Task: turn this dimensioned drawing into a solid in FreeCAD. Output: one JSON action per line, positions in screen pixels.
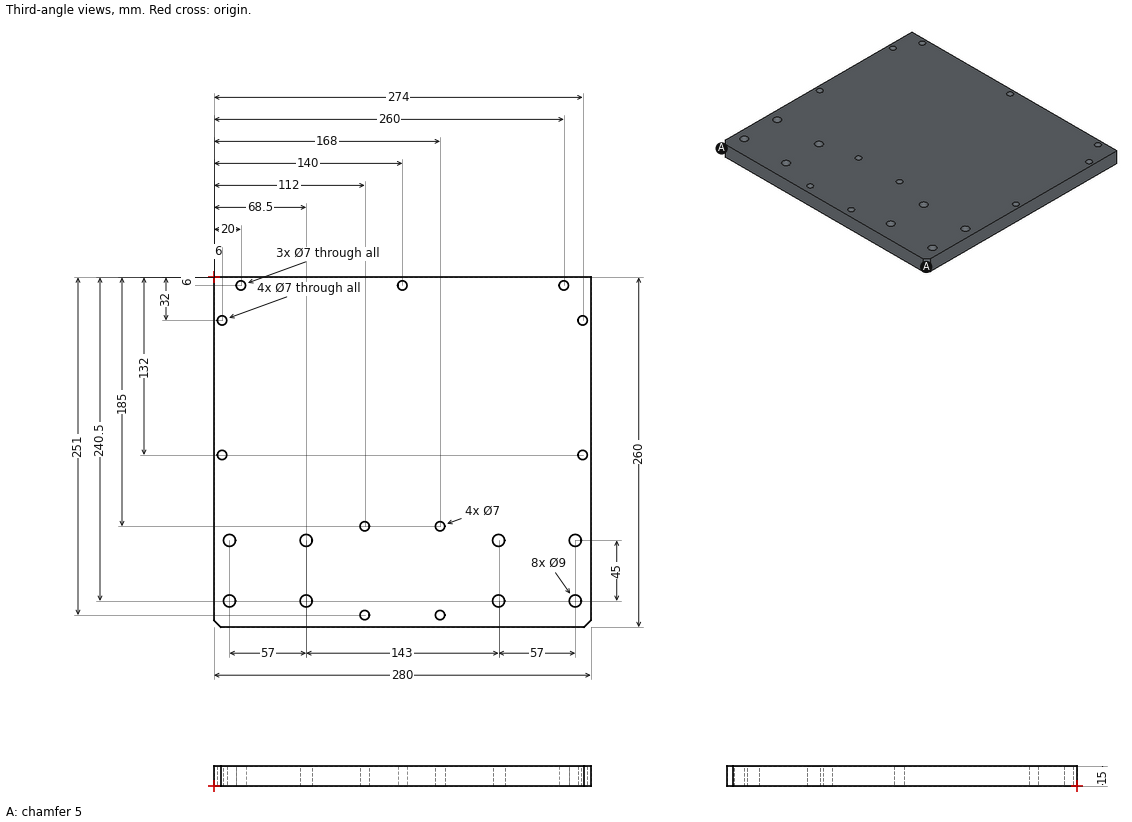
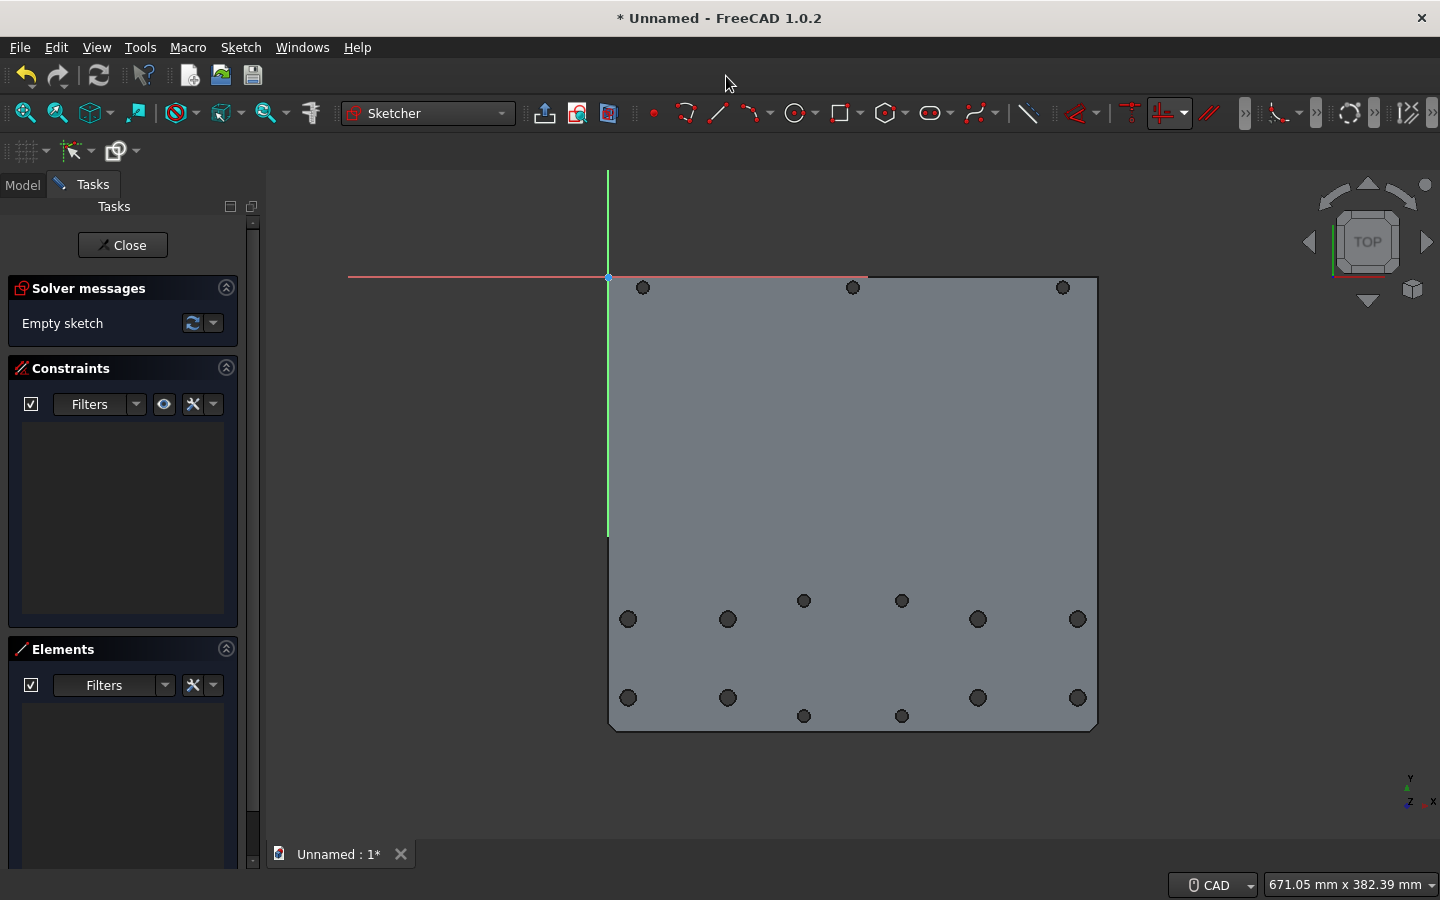
{"action": "scroll", "coordinate": [986, 198], "scroll_direction": "up", "scroll_amount": 2}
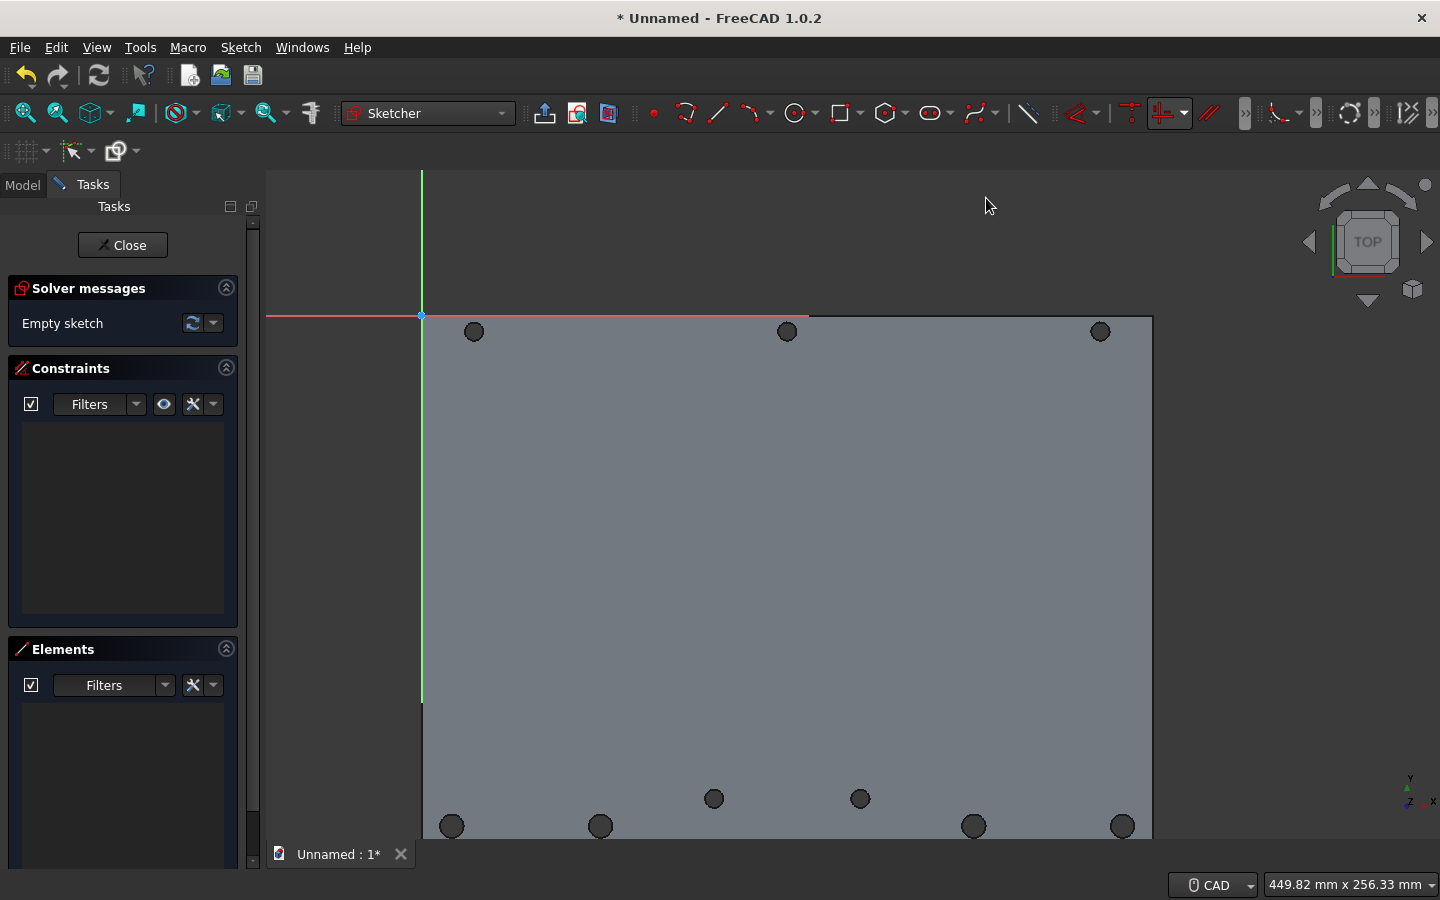
{"action": "left_click", "coordinate": [796, 114]}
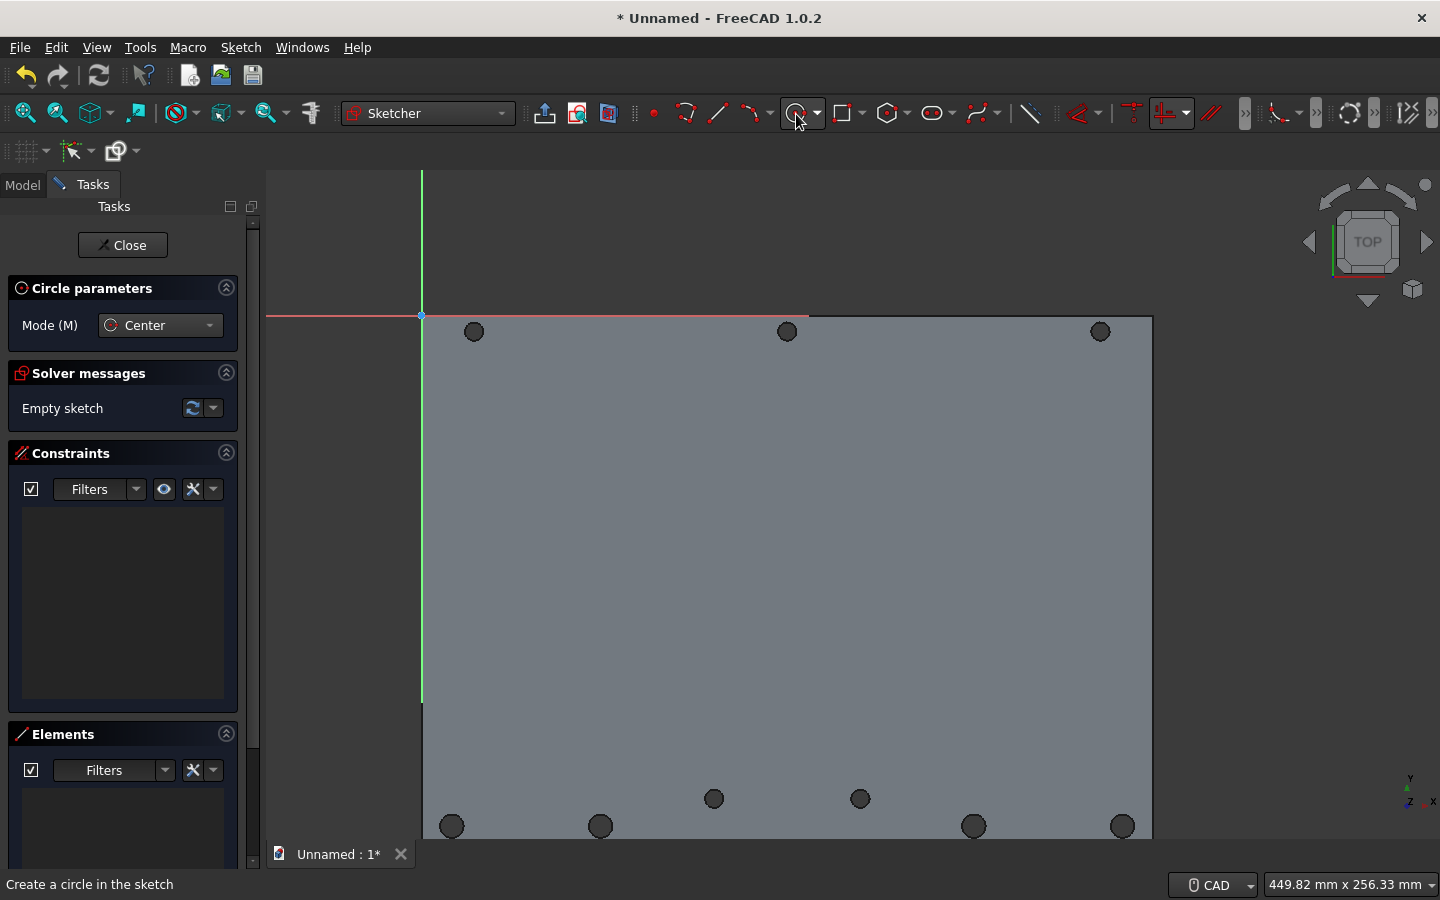
{"action": "scroll", "coordinate": [438, 399], "scroll_direction": "up", "scroll_amount": 5}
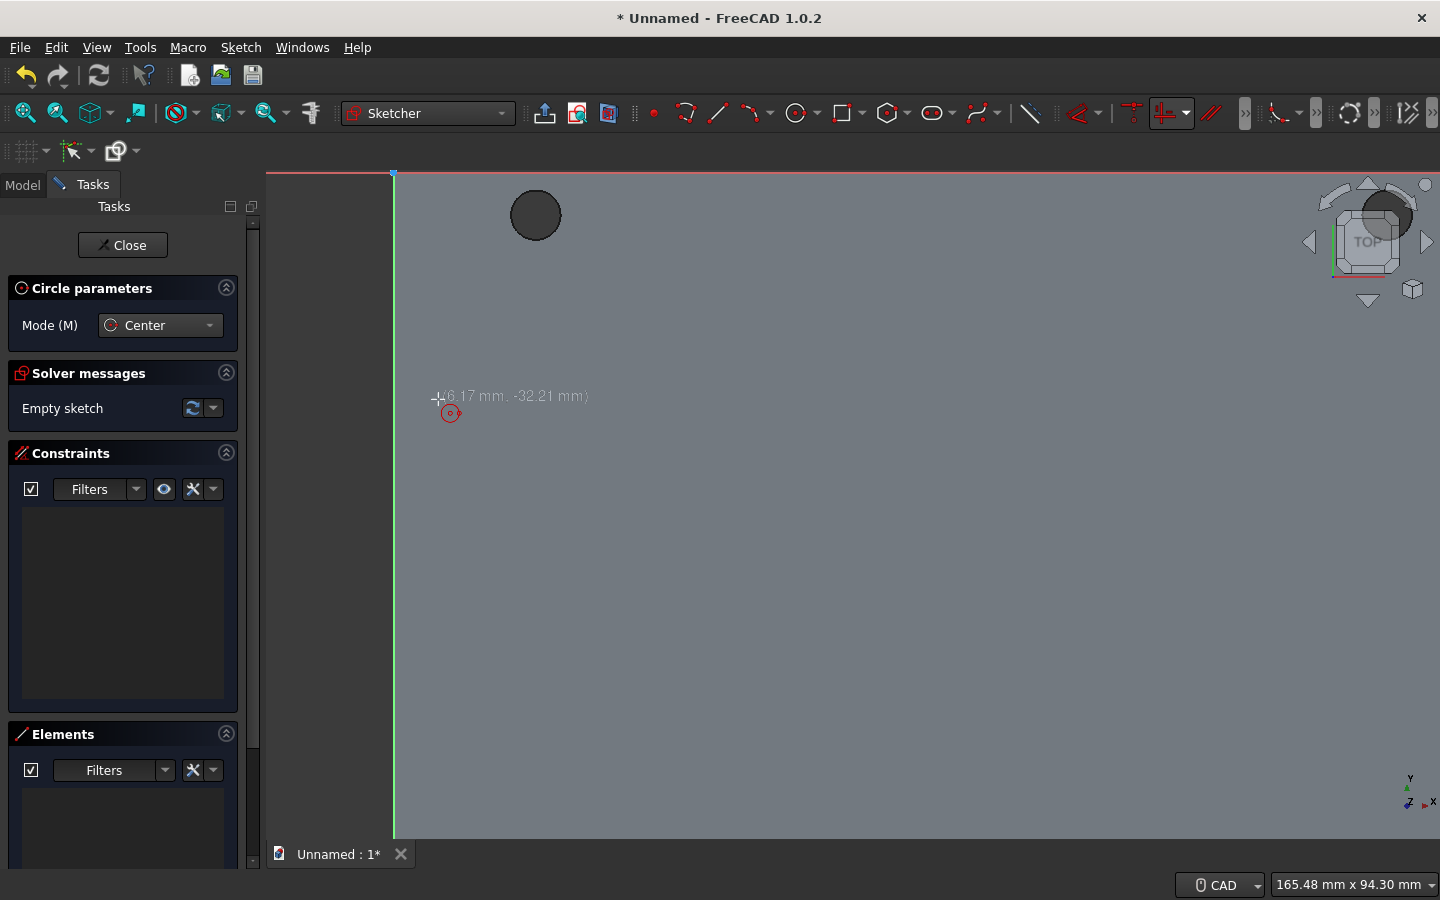
{"action": "left_click", "coordinate": [437, 400]}
{"action": "mouse_move", "coordinate": [454, 382]}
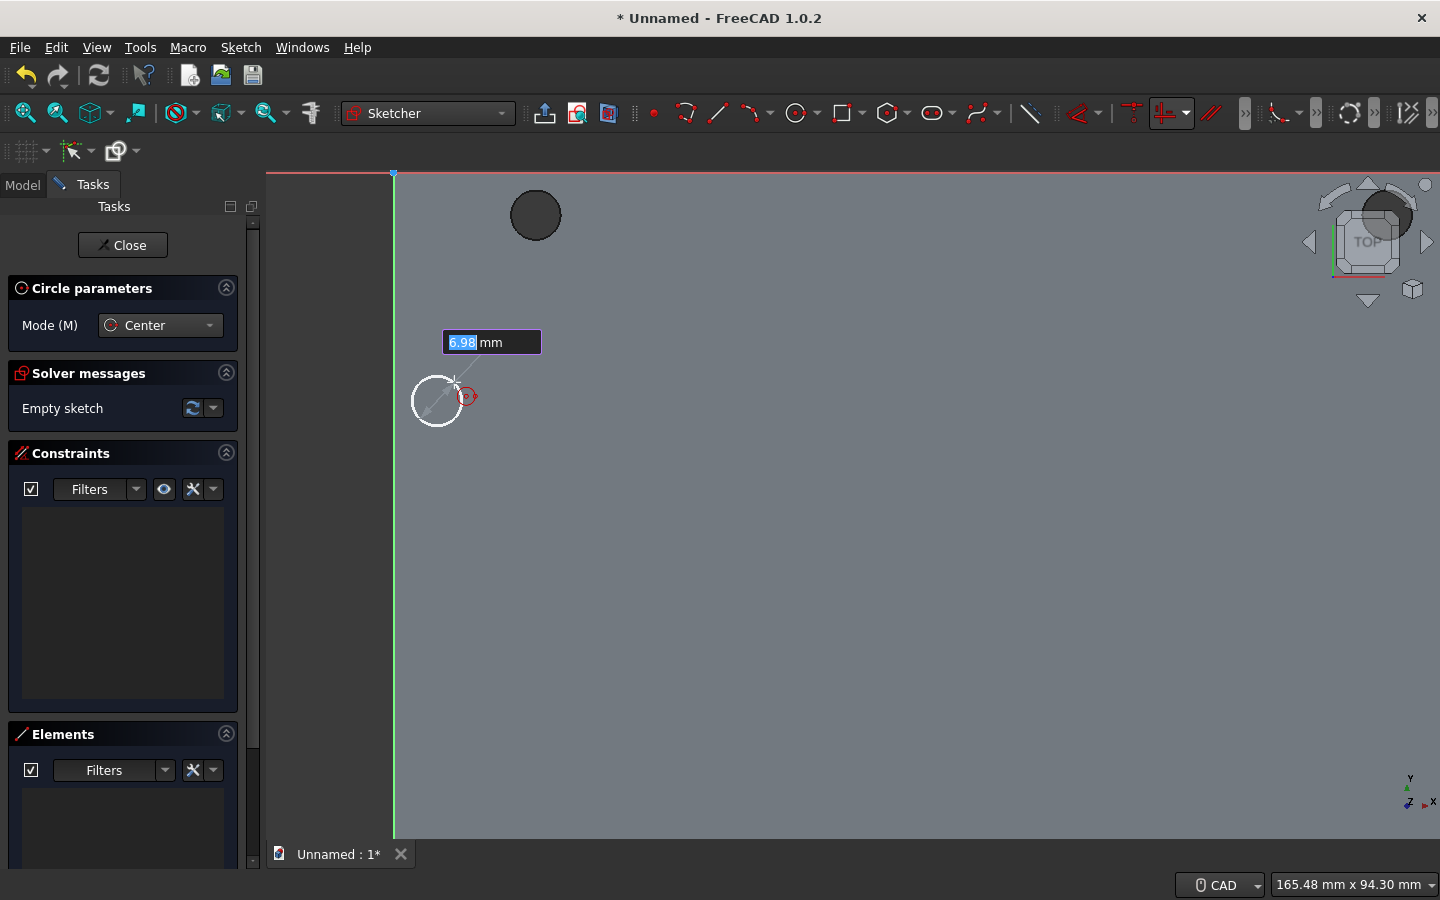
{"action": "type", "text": "7"}
{"action": "key", "text": "Return"}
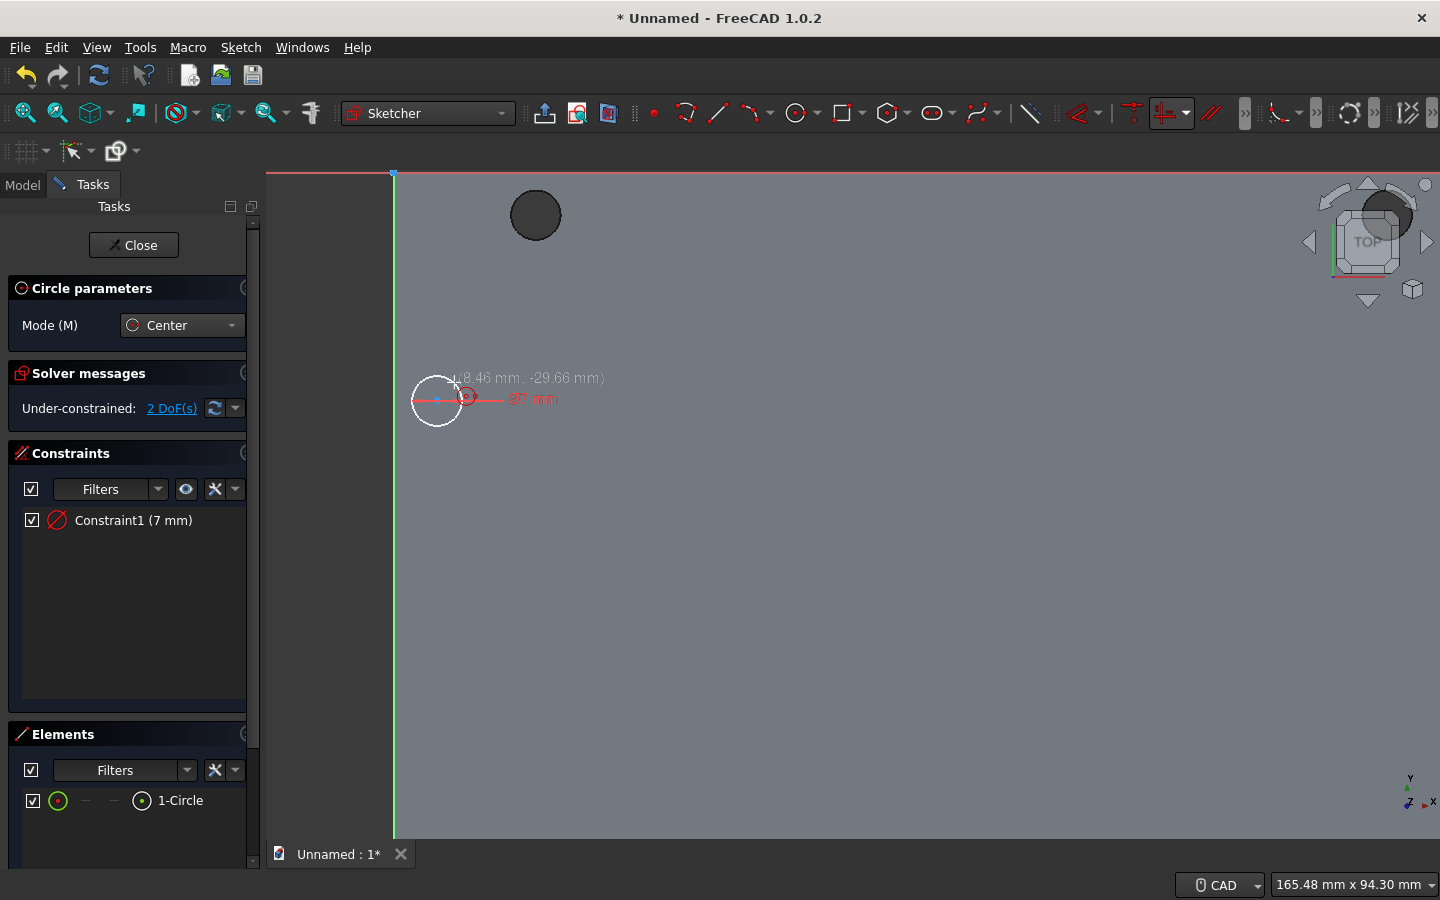
{"action": "scroll", "coordinate": [439, 418], "scroll_direction": "down", "scroll_amount": 5}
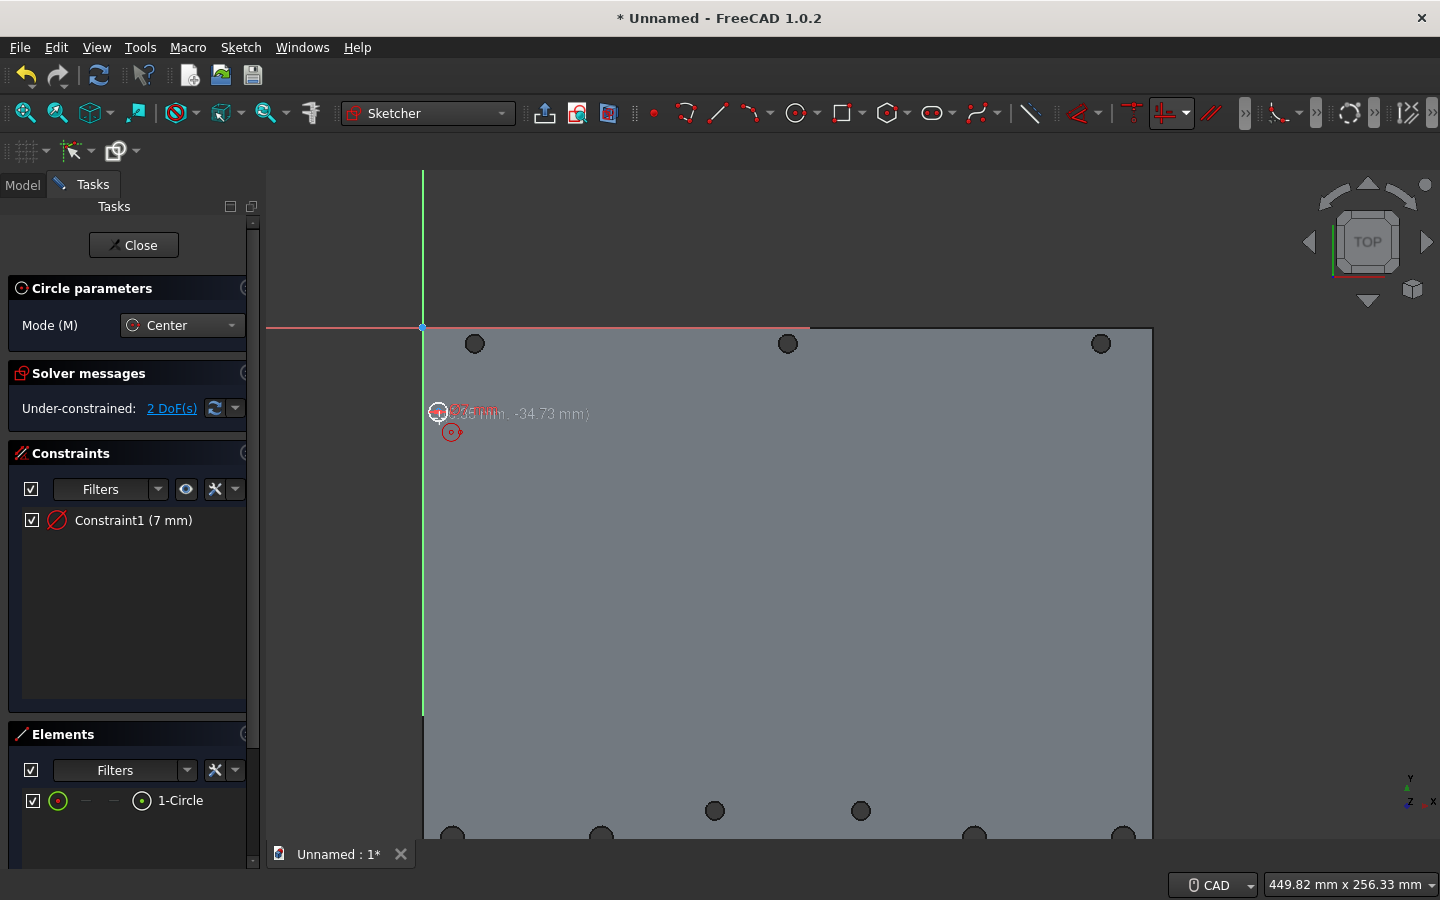
{"action": "scroll", "coordinate": [1138, 411], "scroll_direction": "up", "scroll_amount": 5}